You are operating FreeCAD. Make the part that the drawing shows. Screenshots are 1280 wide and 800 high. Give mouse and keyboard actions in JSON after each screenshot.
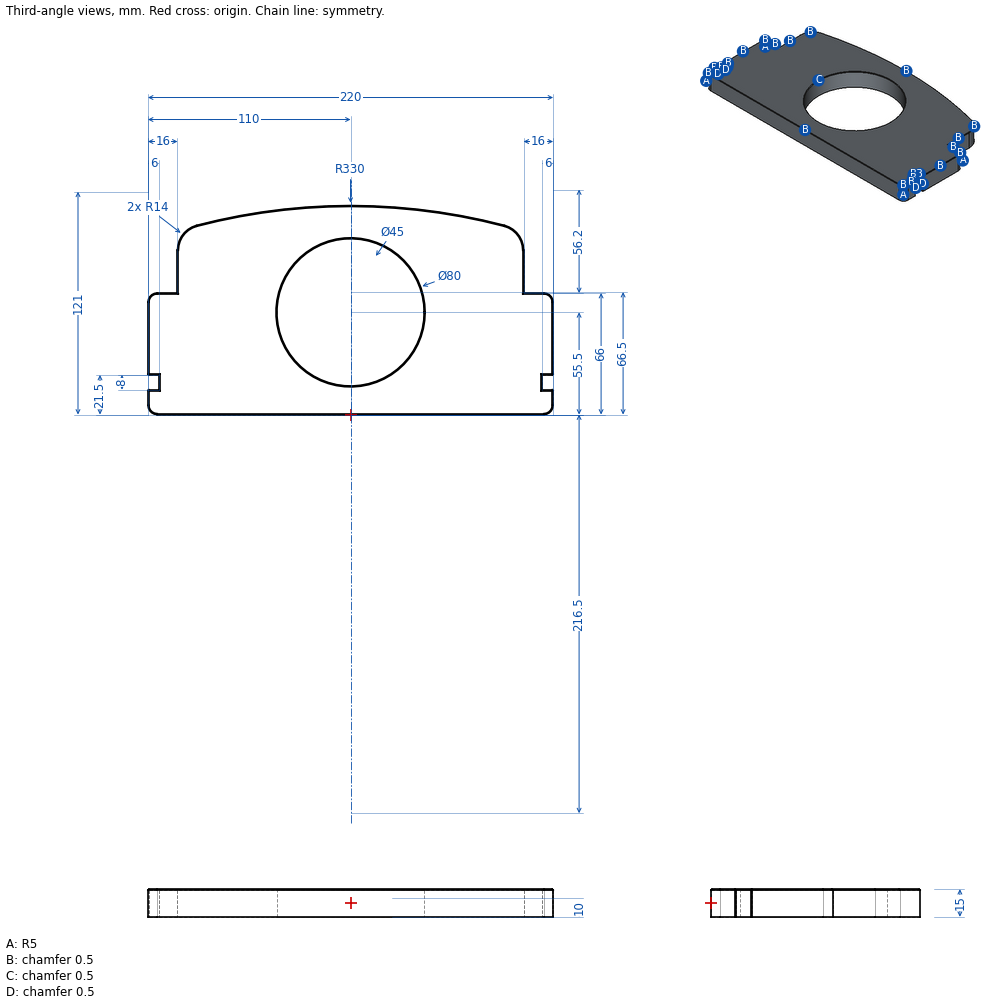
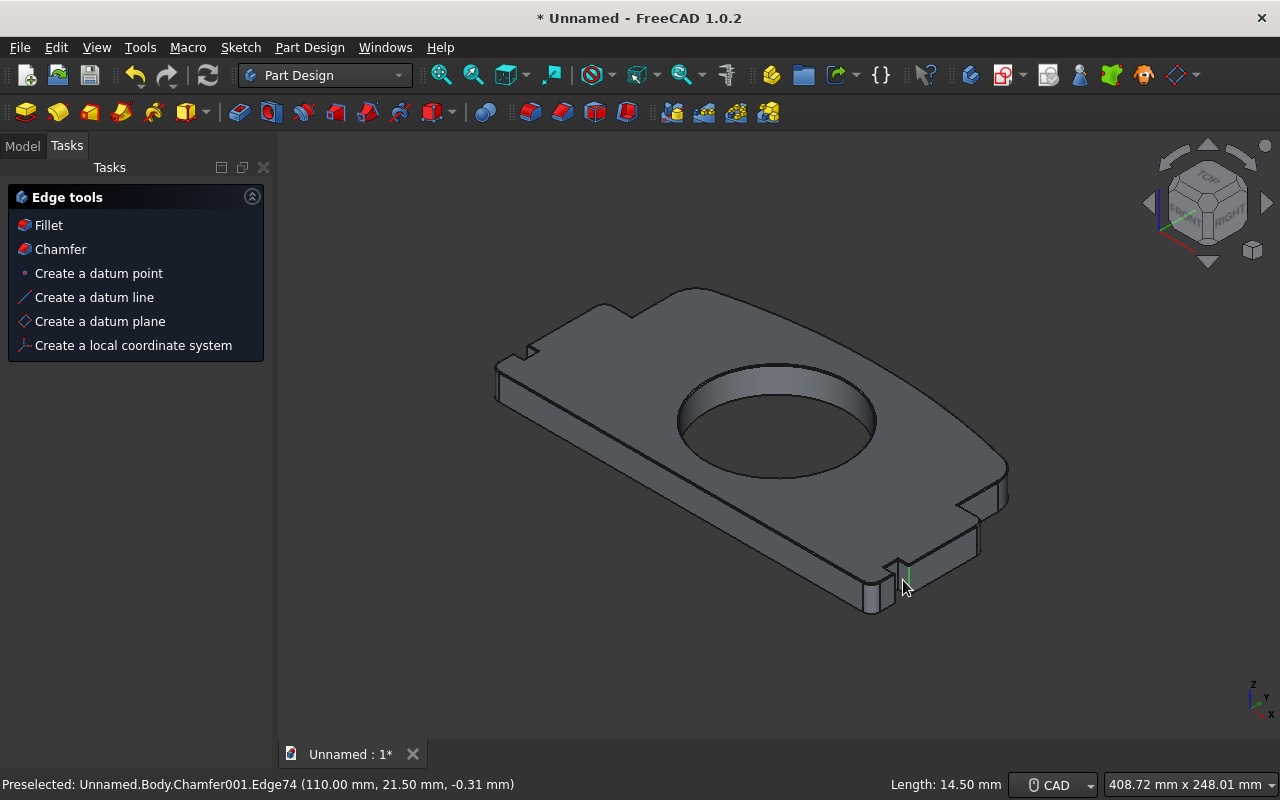
{"action": "key", "text": "0"}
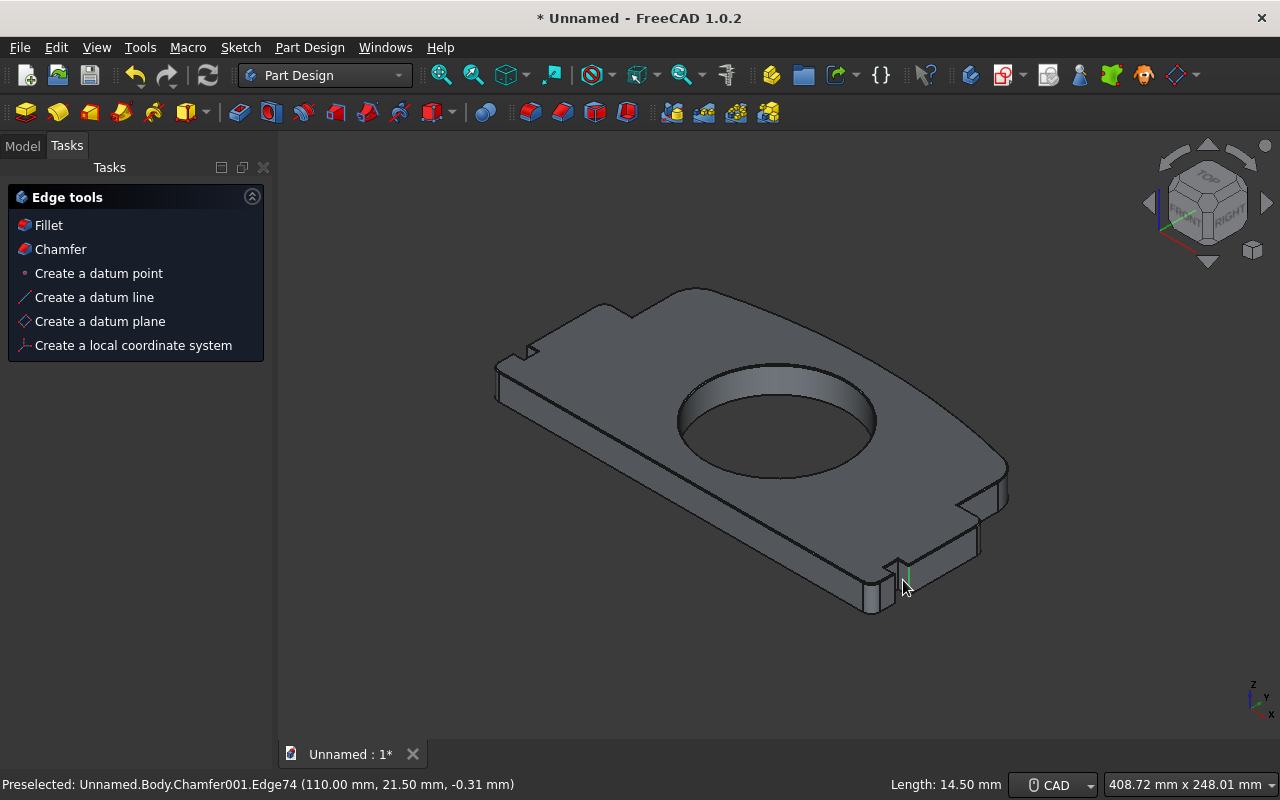
{"action": "key", "text": "1"}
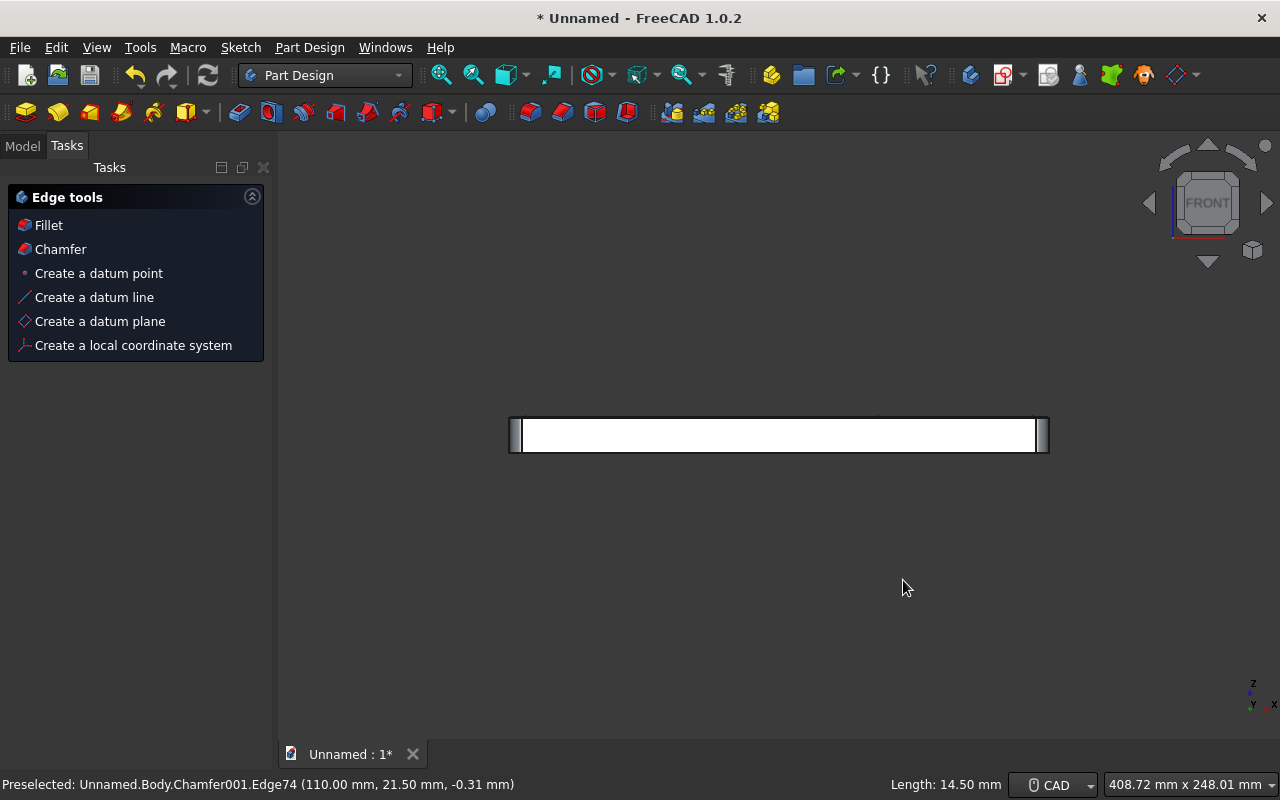
{"action": "key", "text": "3"}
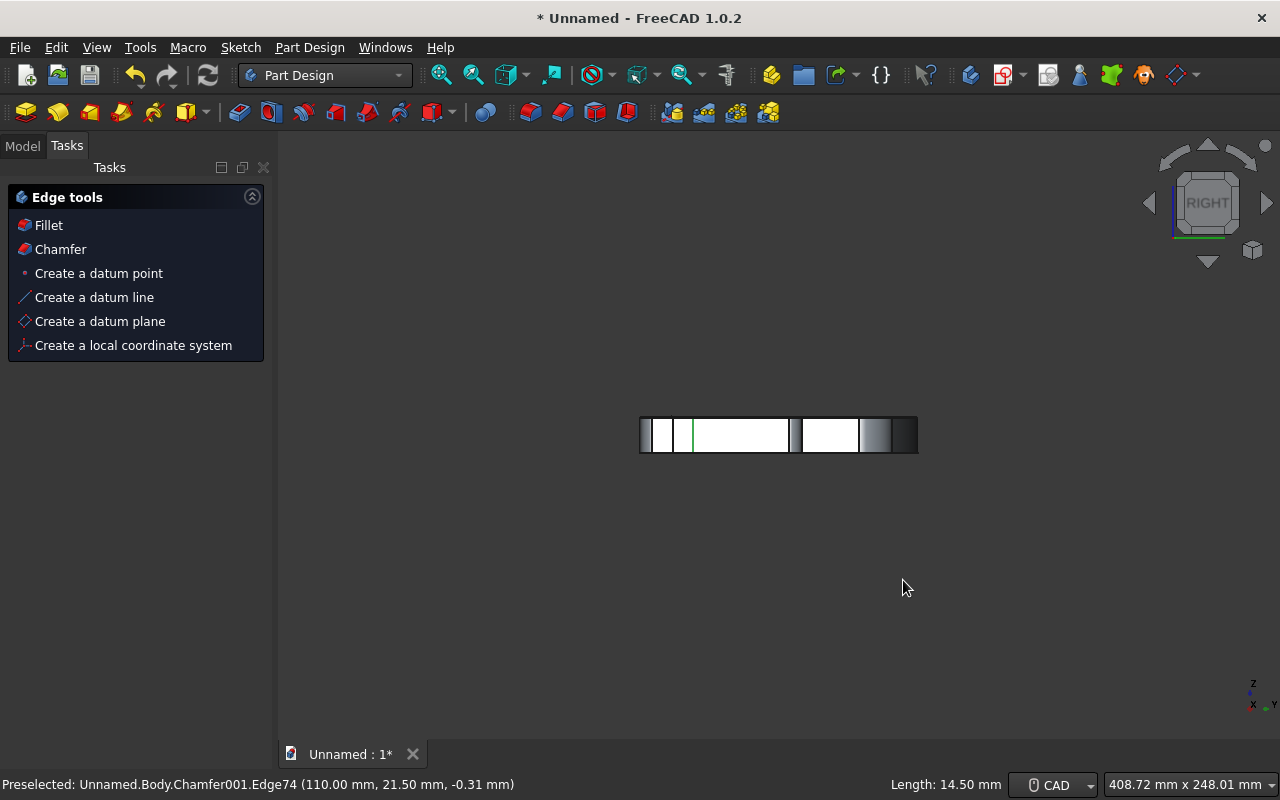
{"action": "left_click", "coordinate": [442, 76]}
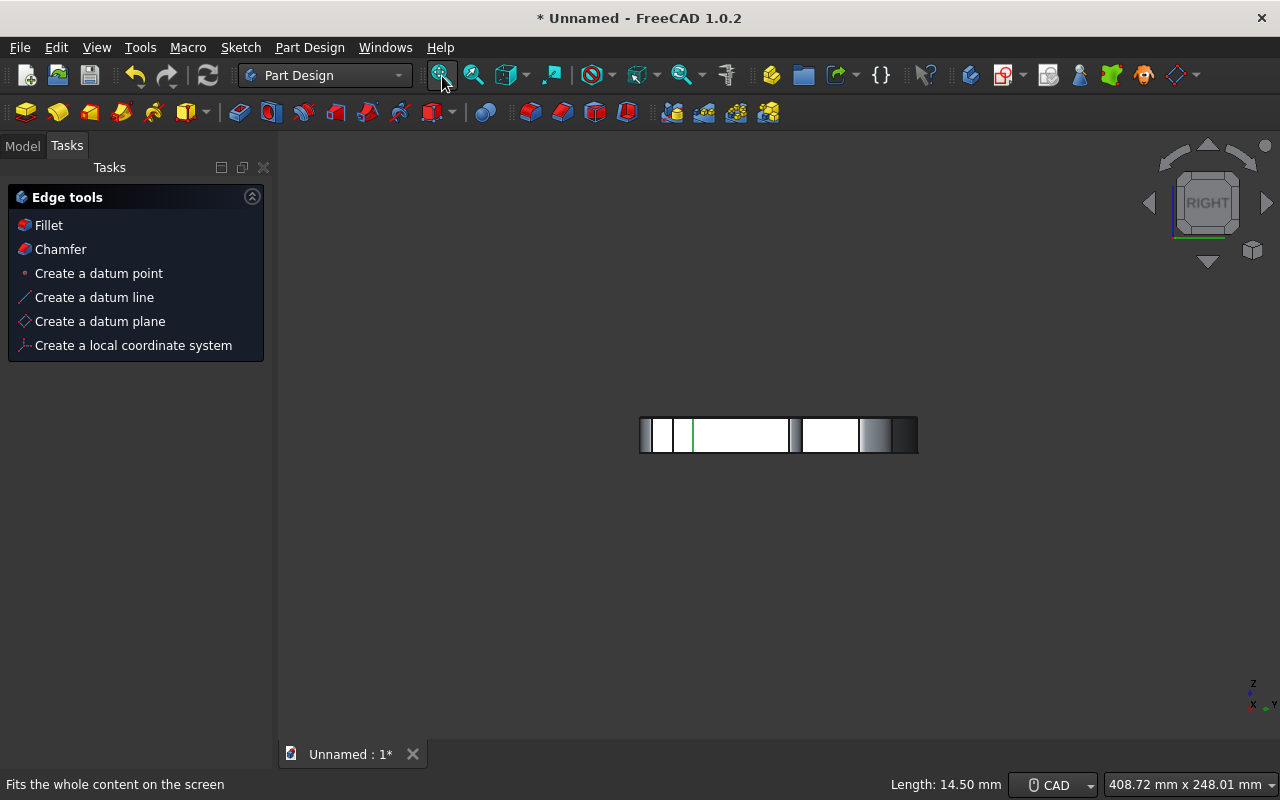
{"action": "left_click", "coordinate": [673, 435], "text": "ctrl"}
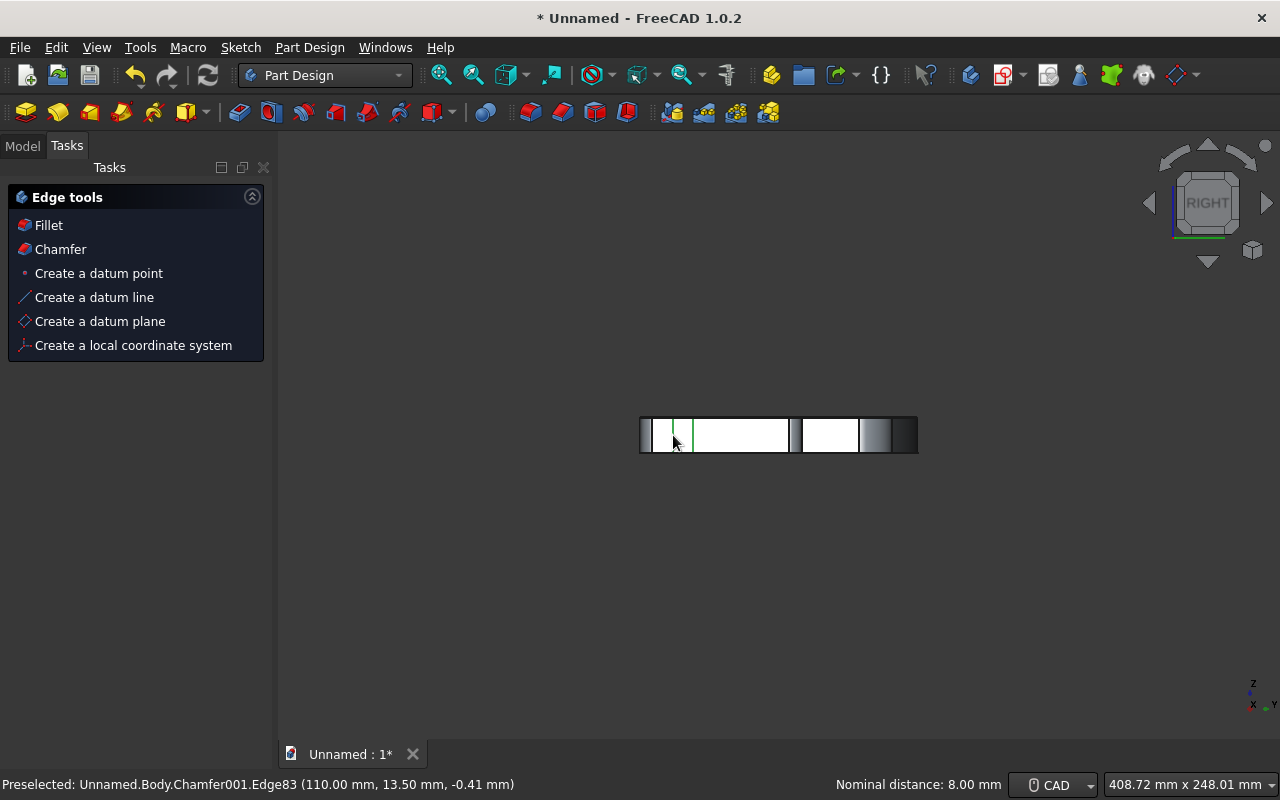
{"action": "key", "text": "5"}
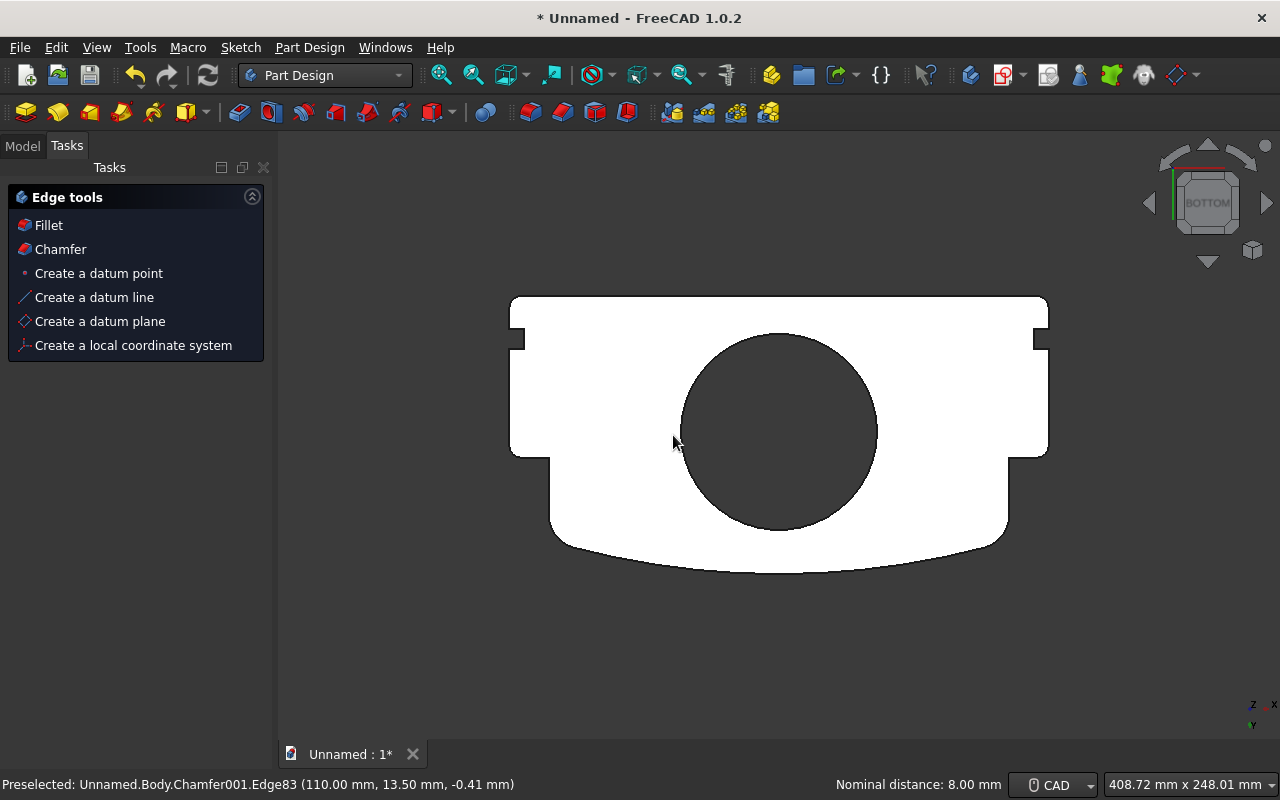
{"action": "key", "text": "4"}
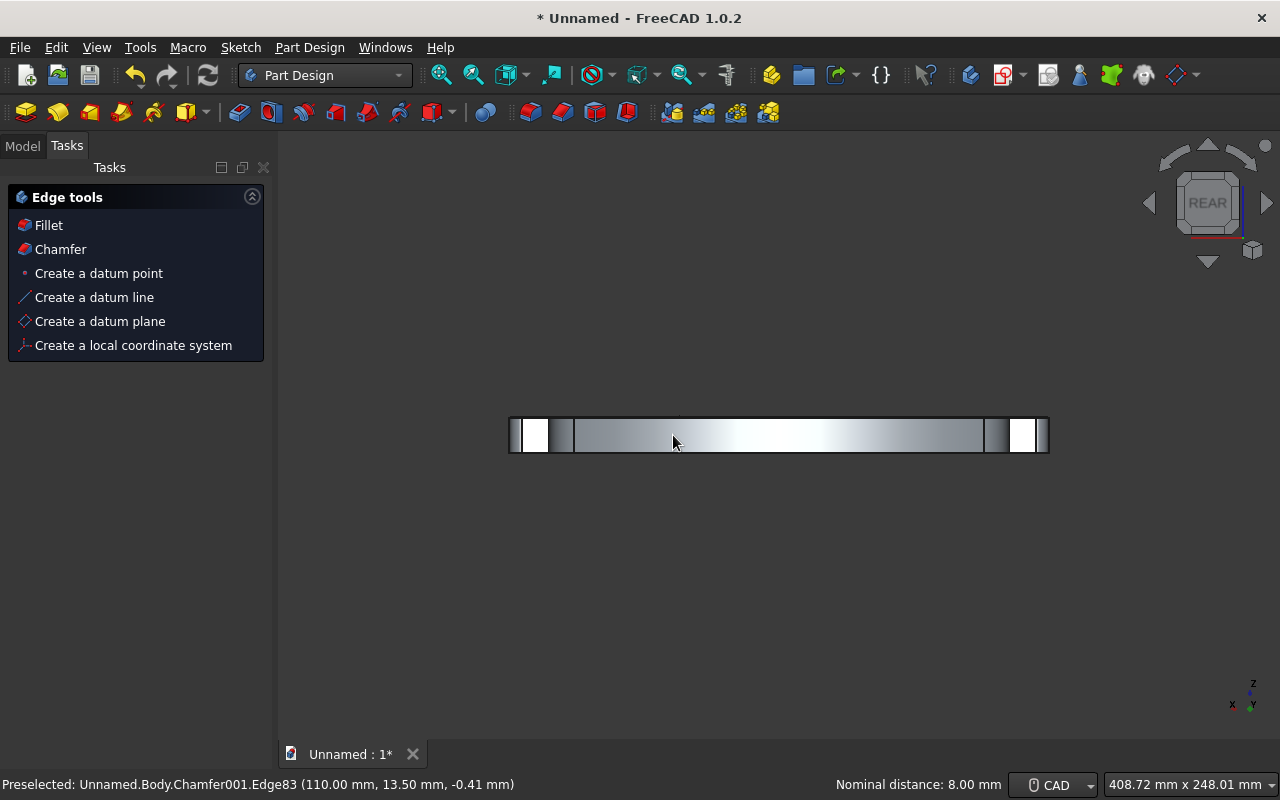
{"action": "key", "text": "6"}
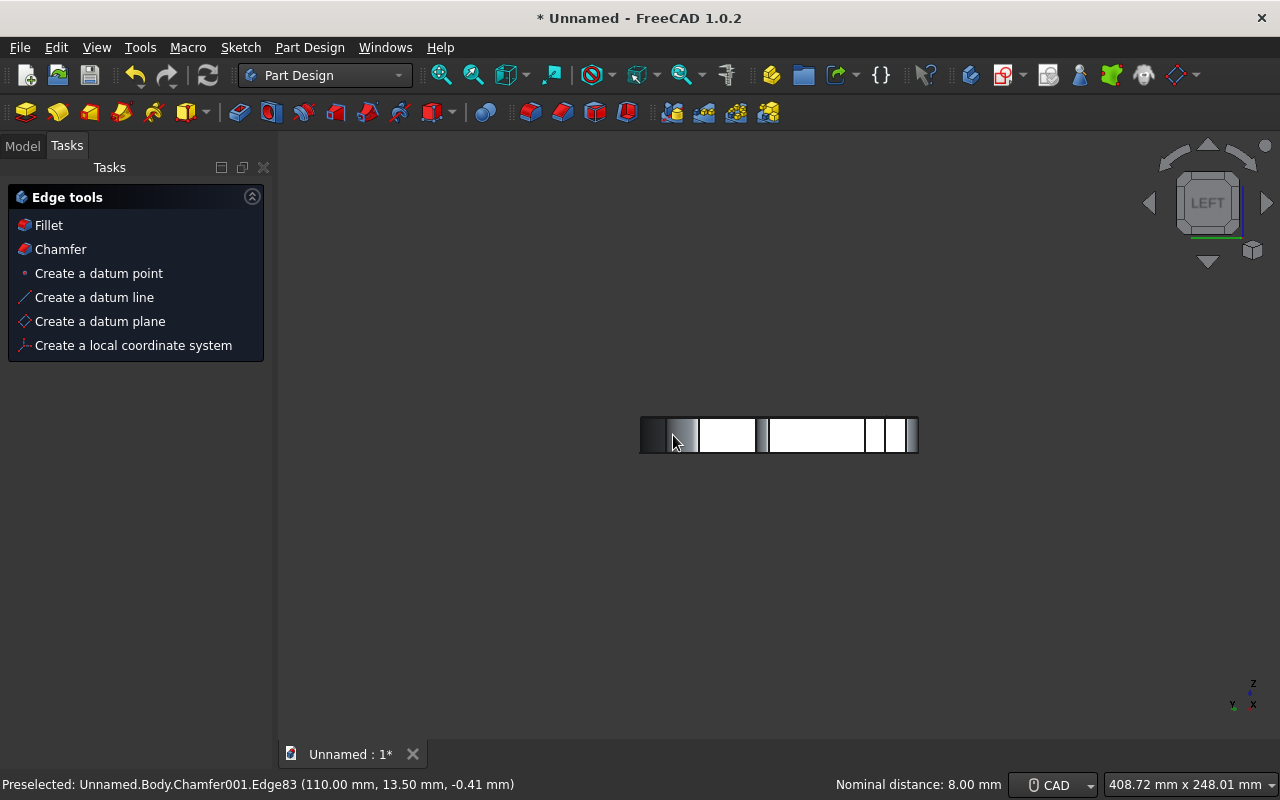
{"action": "left_click", "coordinate": [442, 76]}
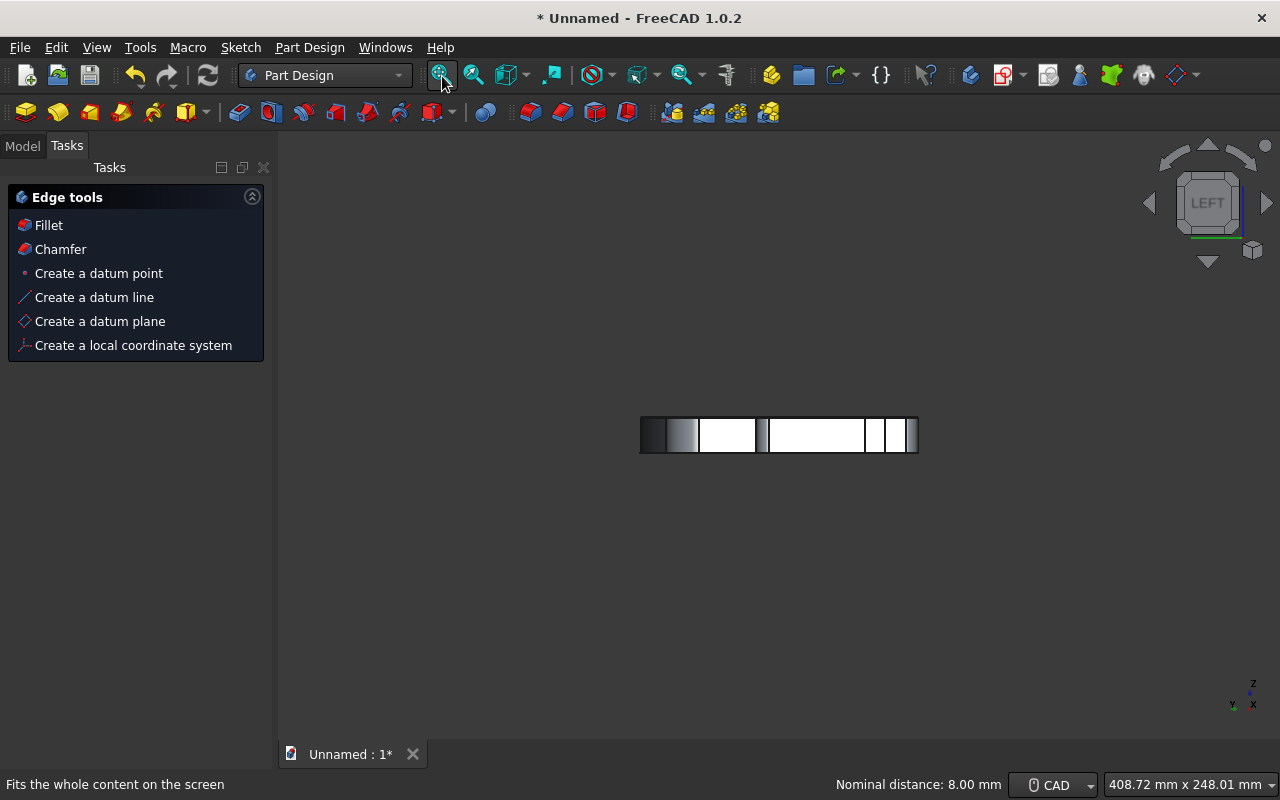
{"action": "left_click", "coordinate": [885, 435], "text": "ctrl"}